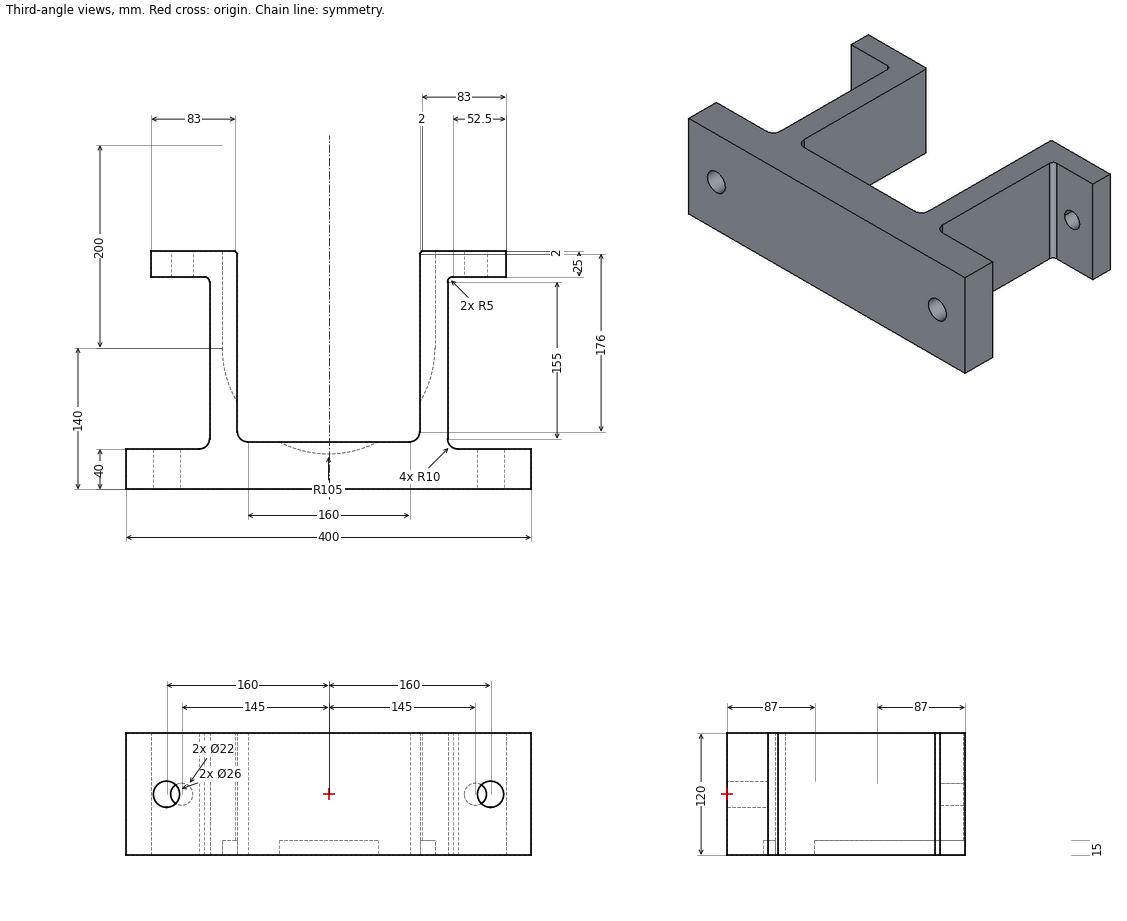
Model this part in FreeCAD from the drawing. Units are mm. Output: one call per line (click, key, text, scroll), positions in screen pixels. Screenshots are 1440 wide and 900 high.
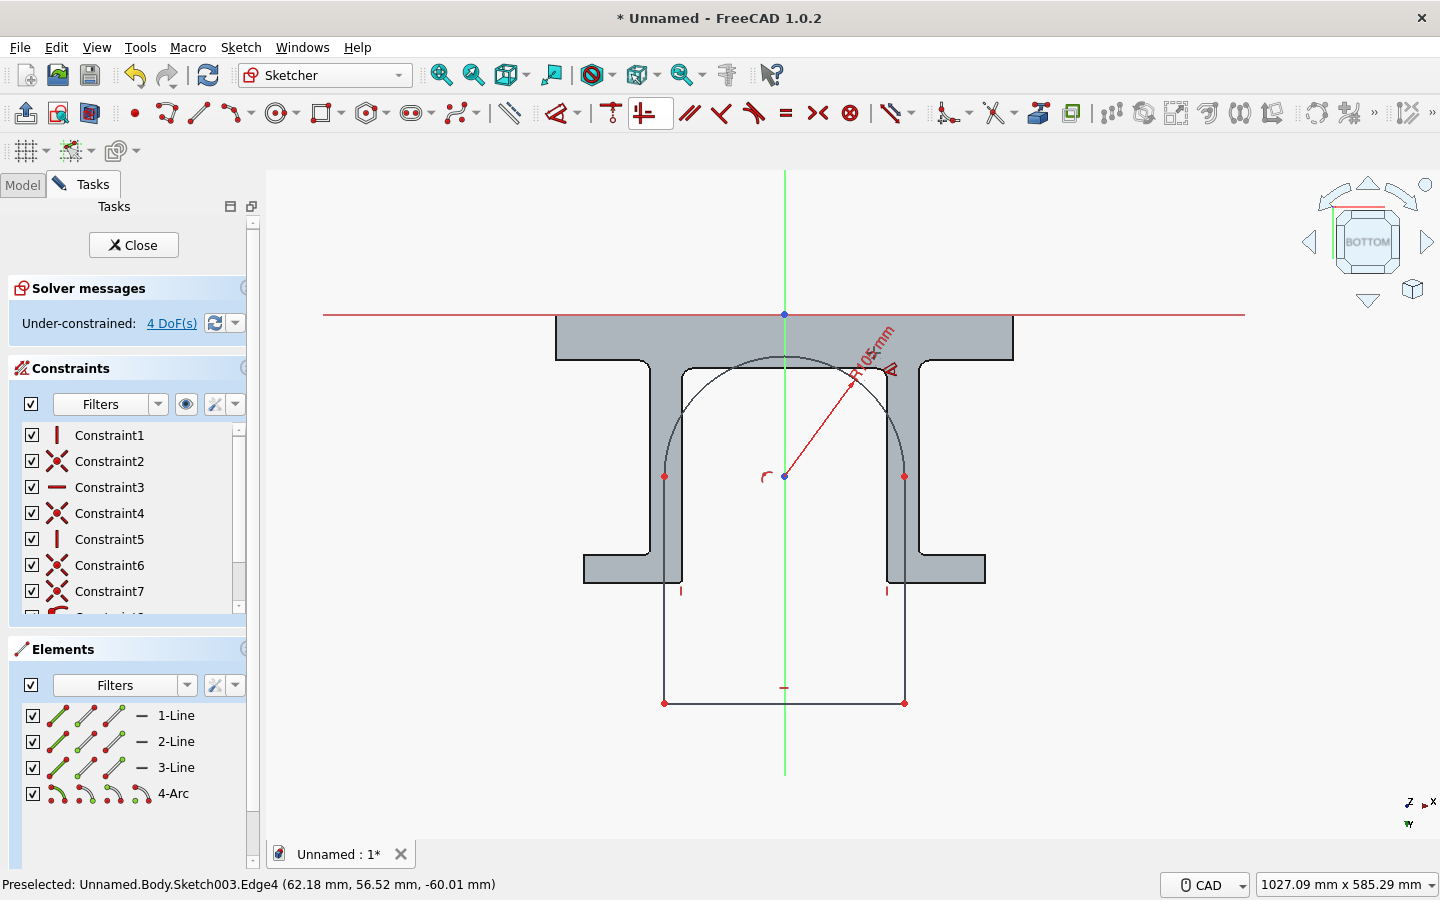
click(664, 544)
click(630, 590)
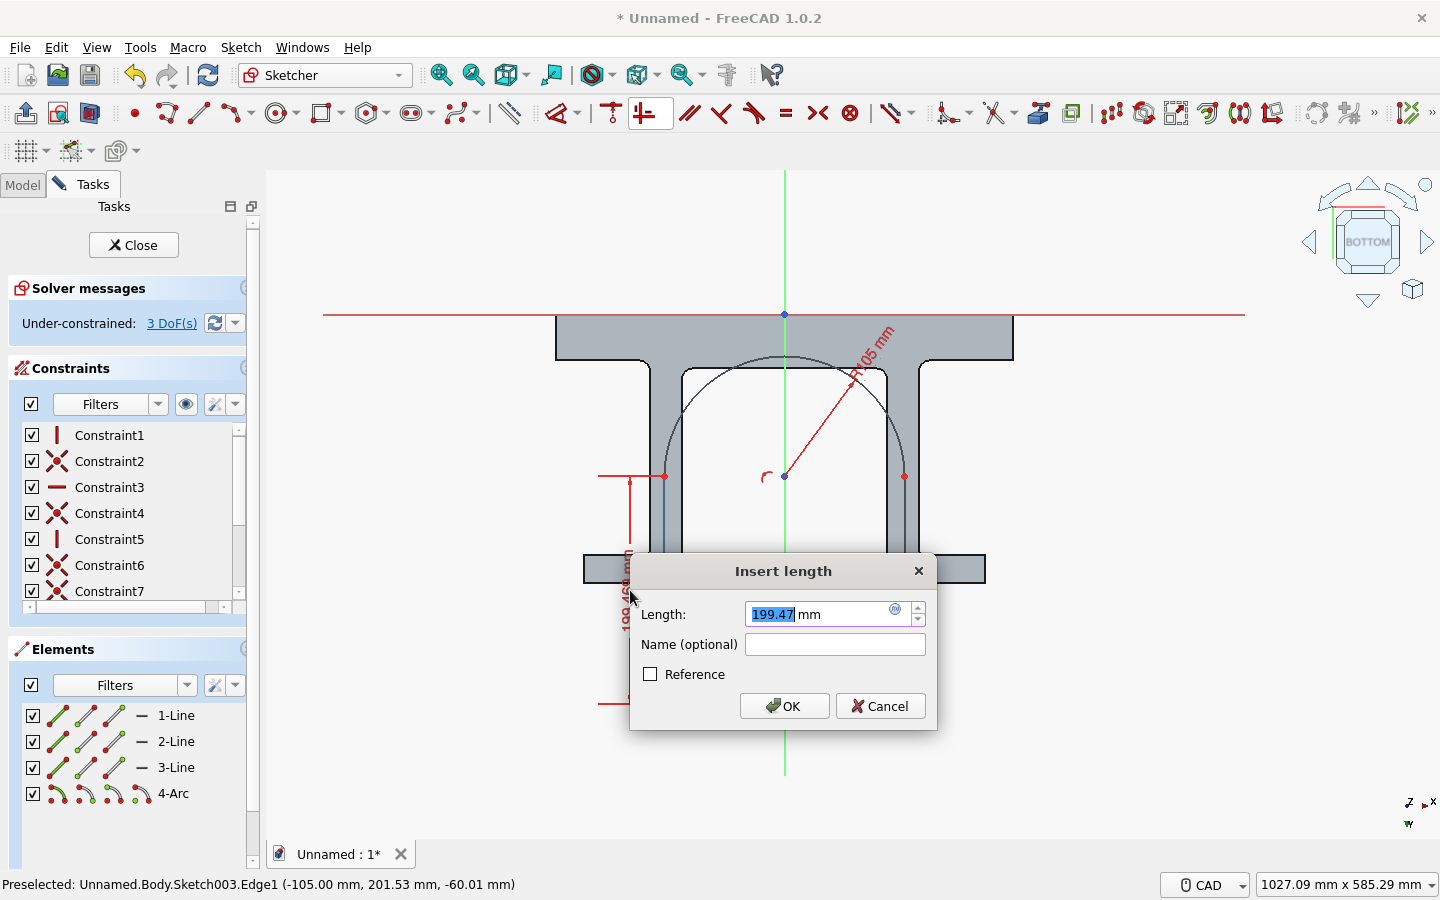
text(200)
key(Return)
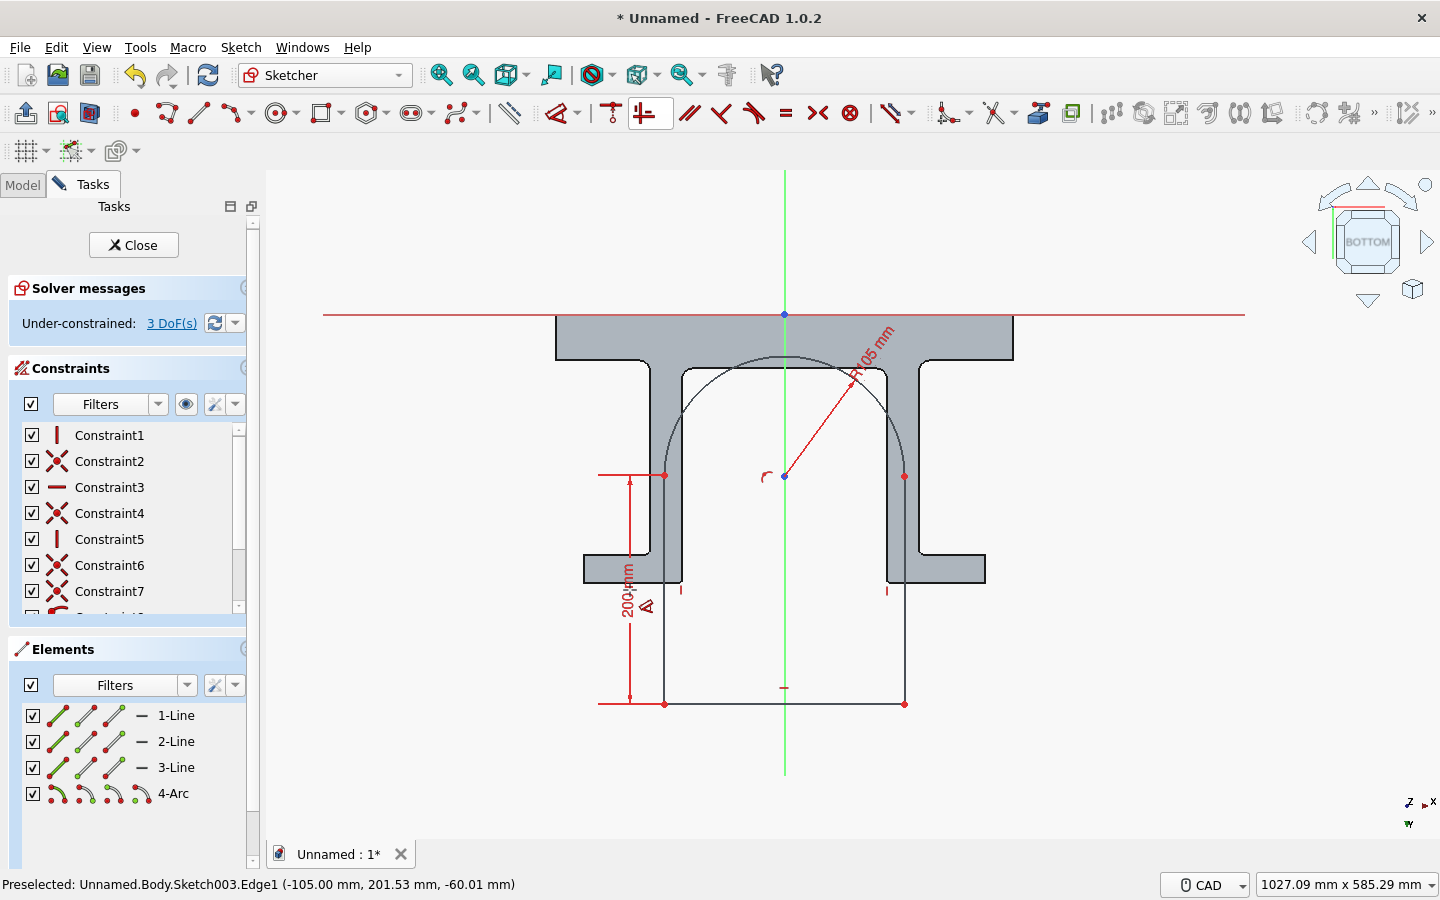
click(905, 636)
click(939, 590)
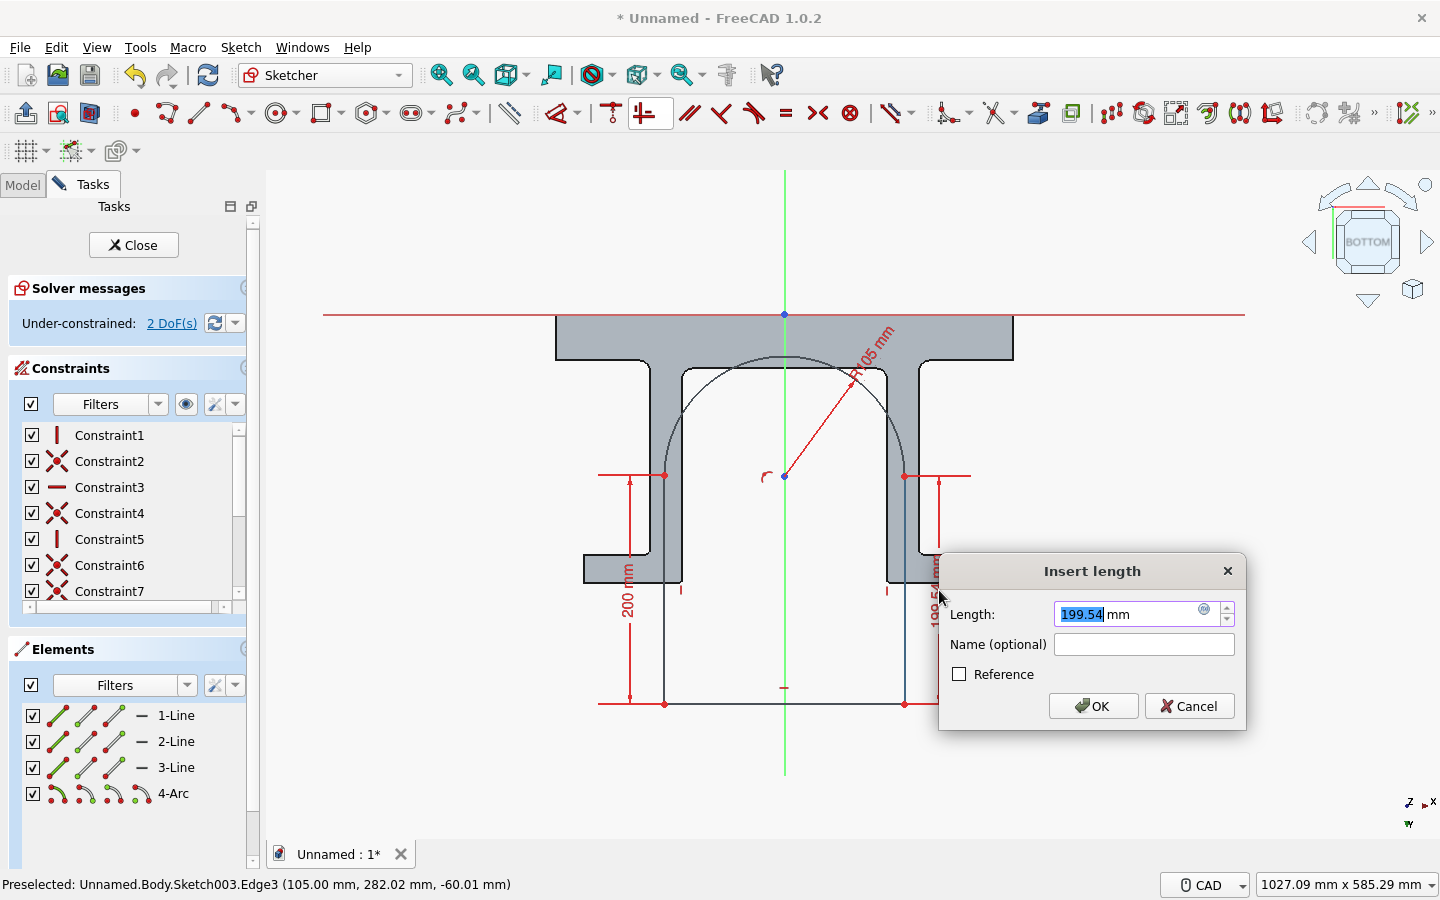
text(200)
key(Return)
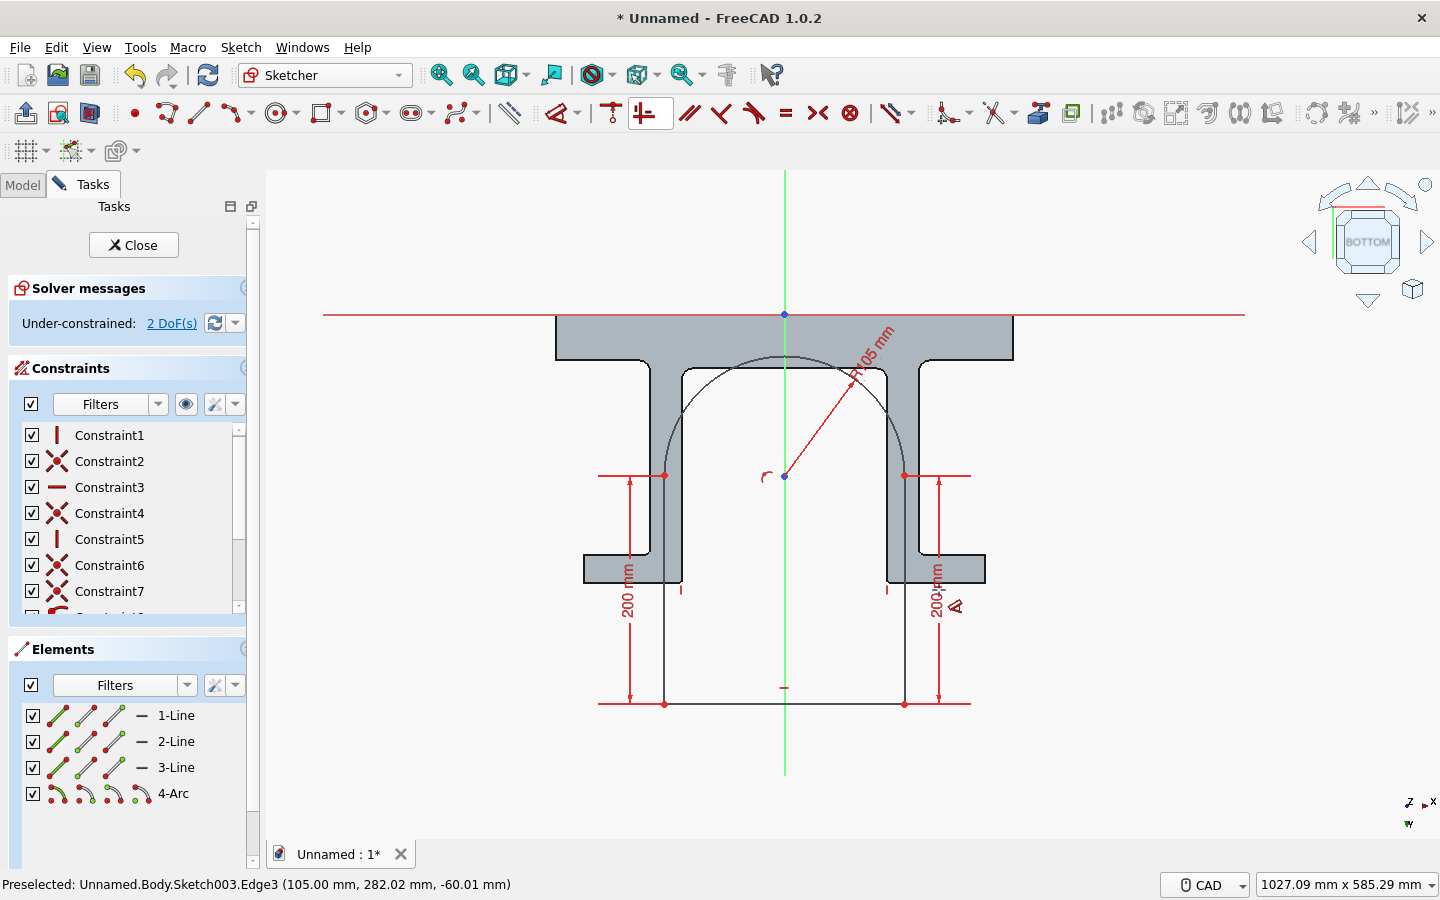
click(664, 476)
click(630, 395)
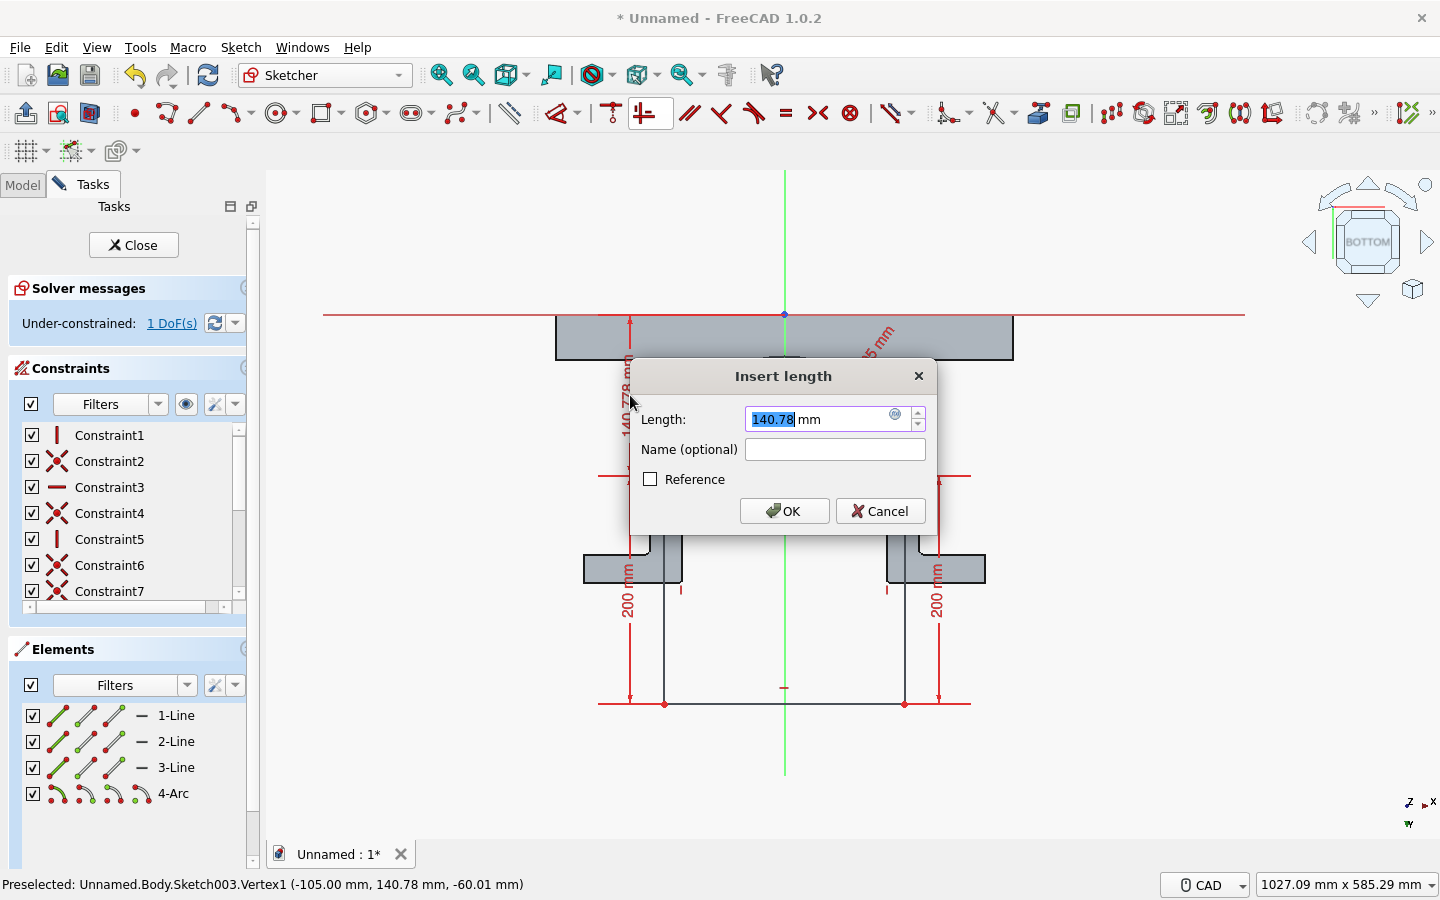
text(140)
key(Return)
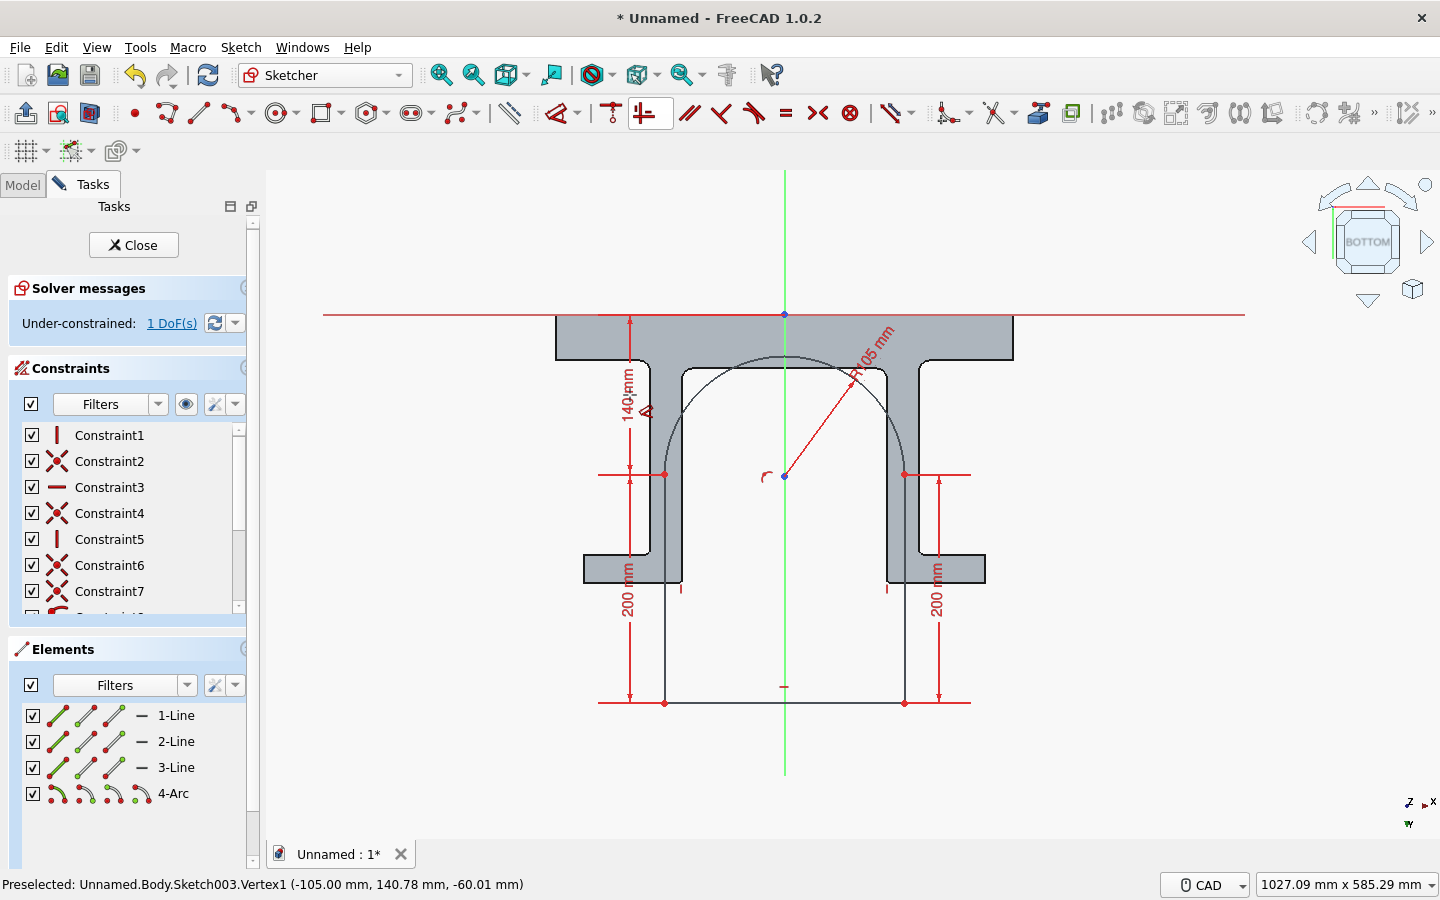
click(785, 477)
click(819, 396)